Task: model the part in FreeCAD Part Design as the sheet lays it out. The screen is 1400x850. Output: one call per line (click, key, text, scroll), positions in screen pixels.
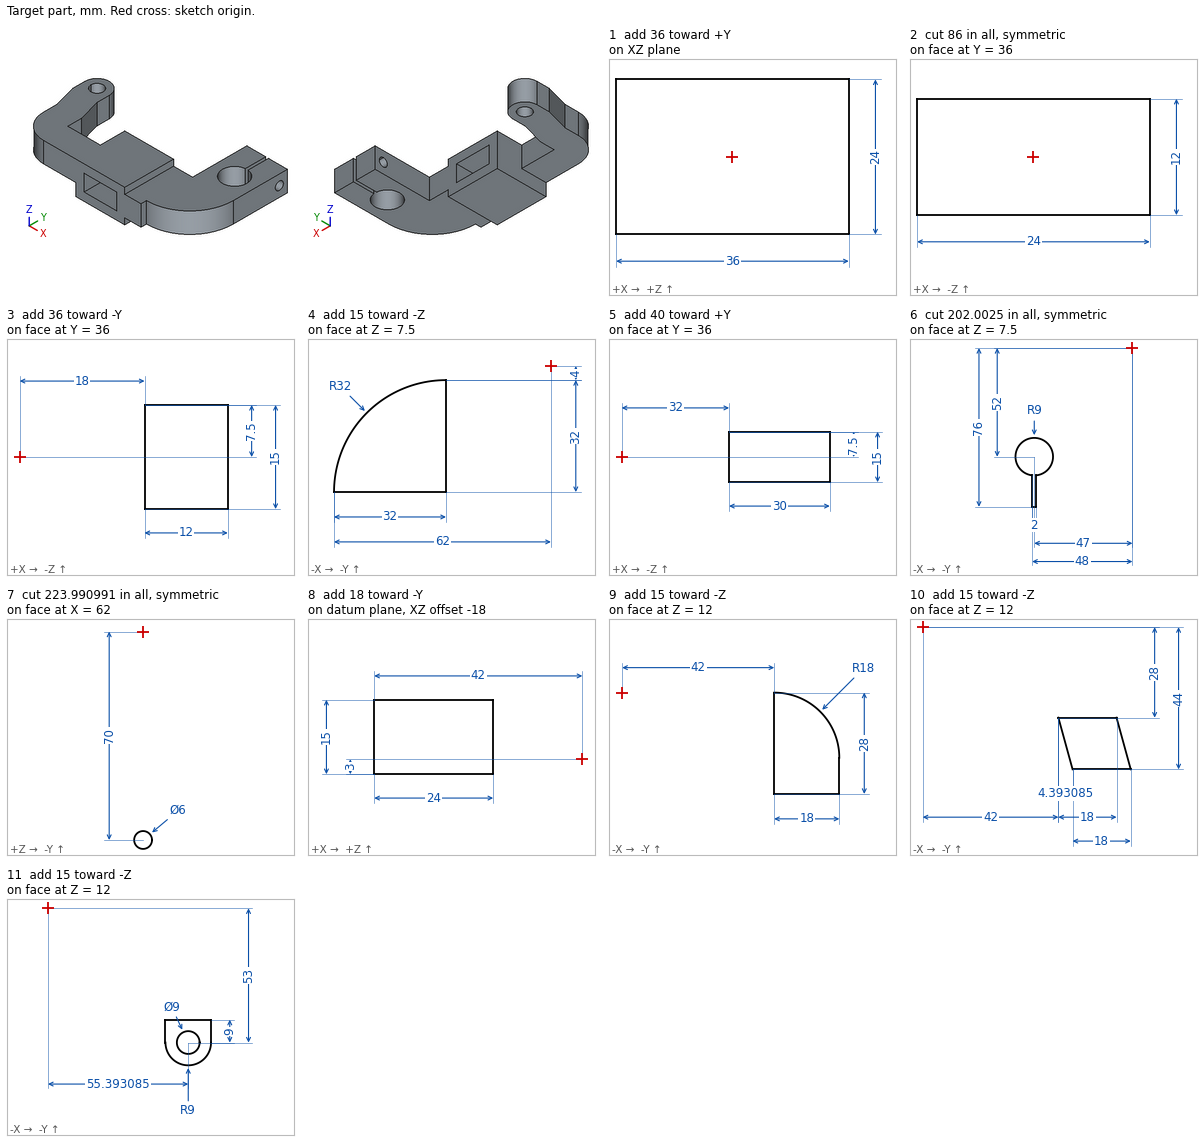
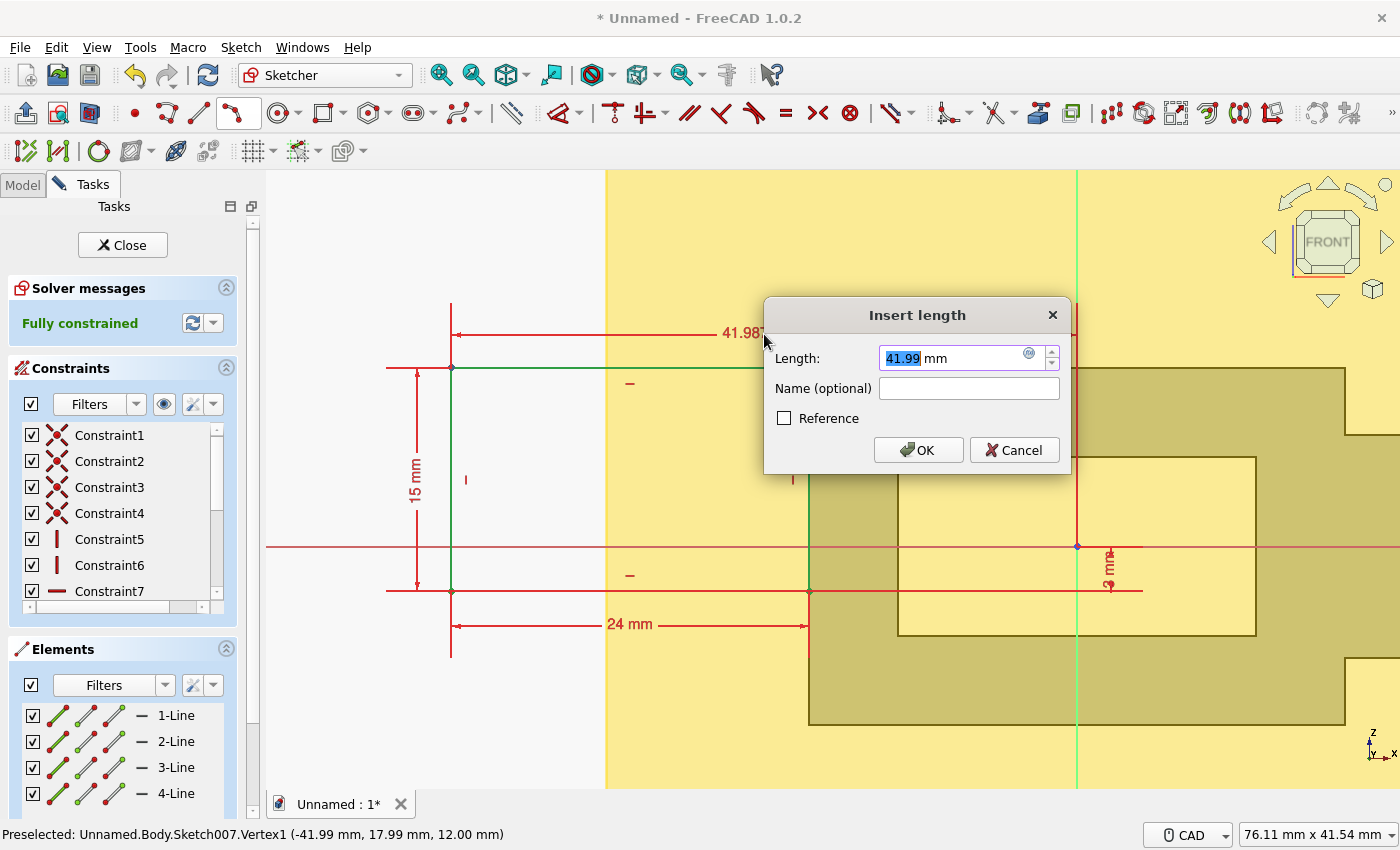
text(42)
key(Return)
key(Escape)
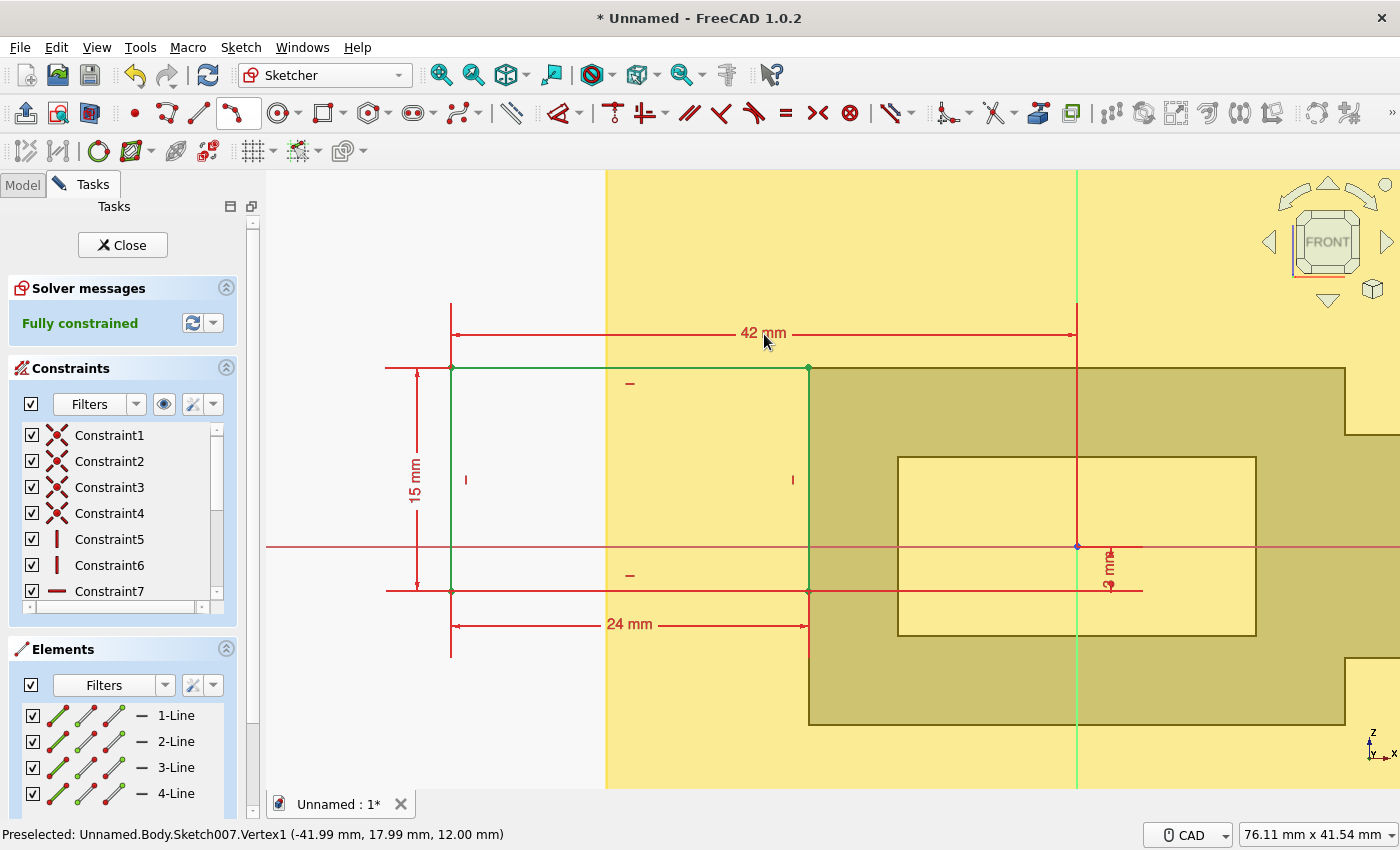
click(123, 245)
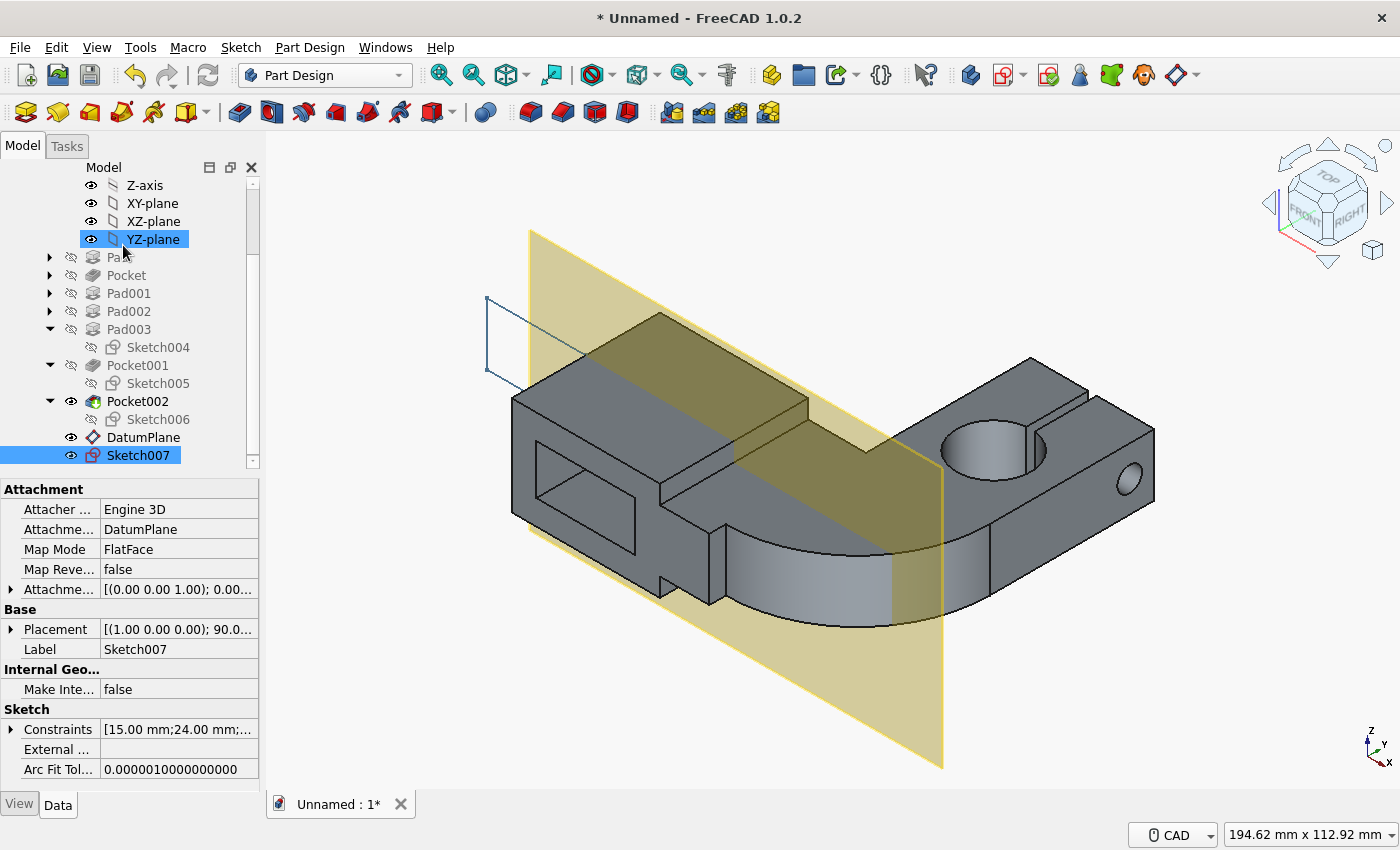
click(26, 112)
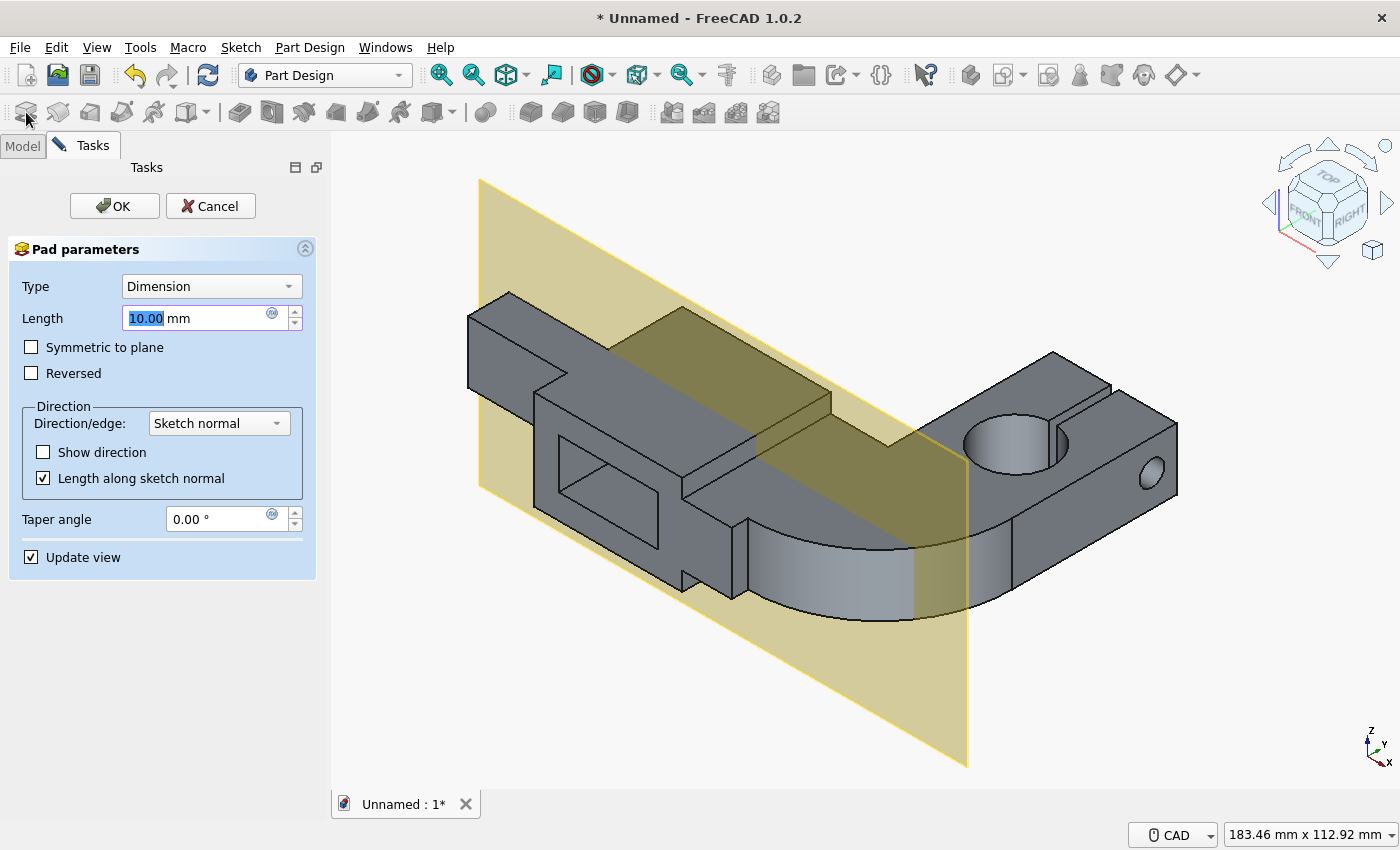
text(18)
key(Tab)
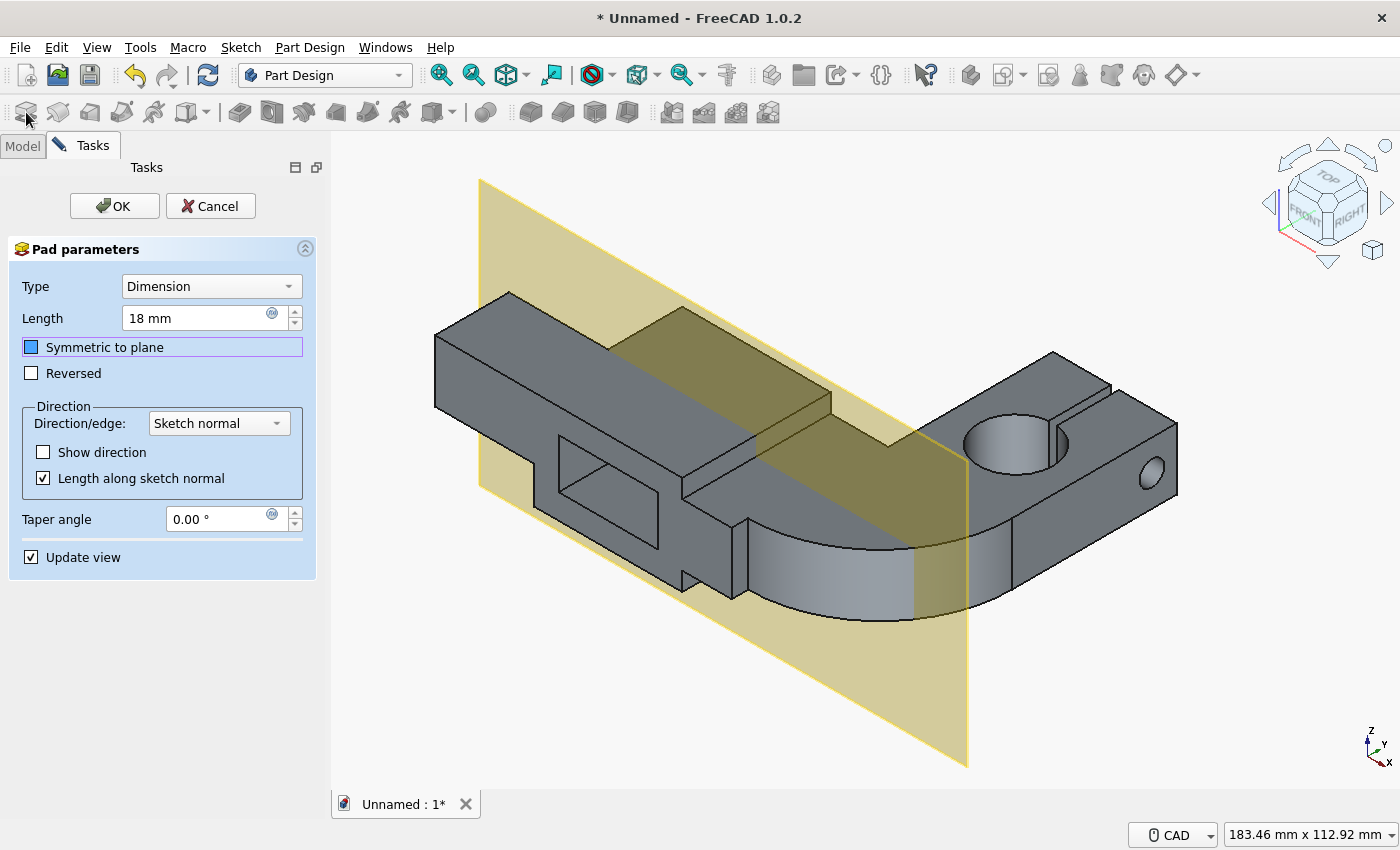
click(115, 206)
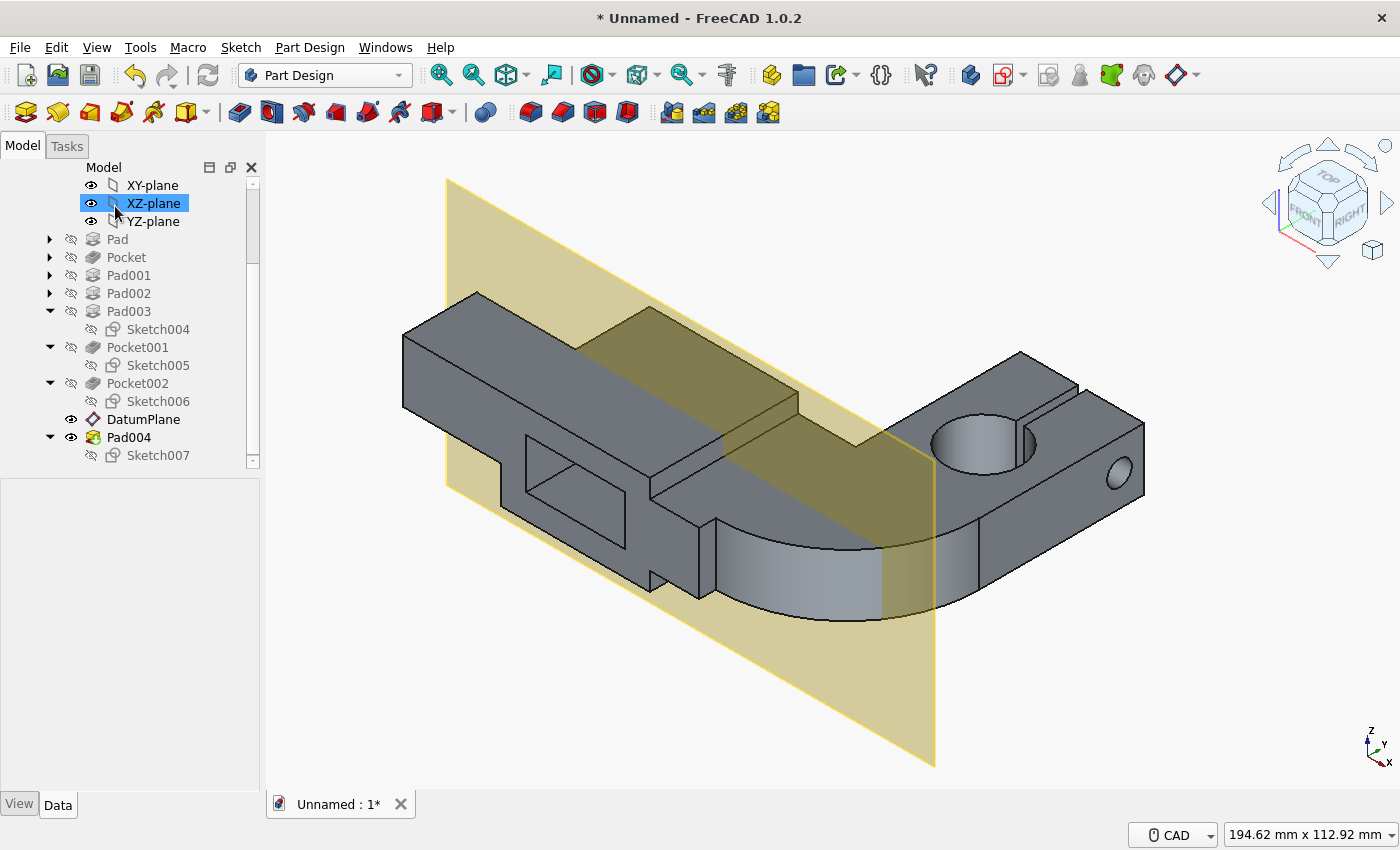
click(116, 419)
key(space)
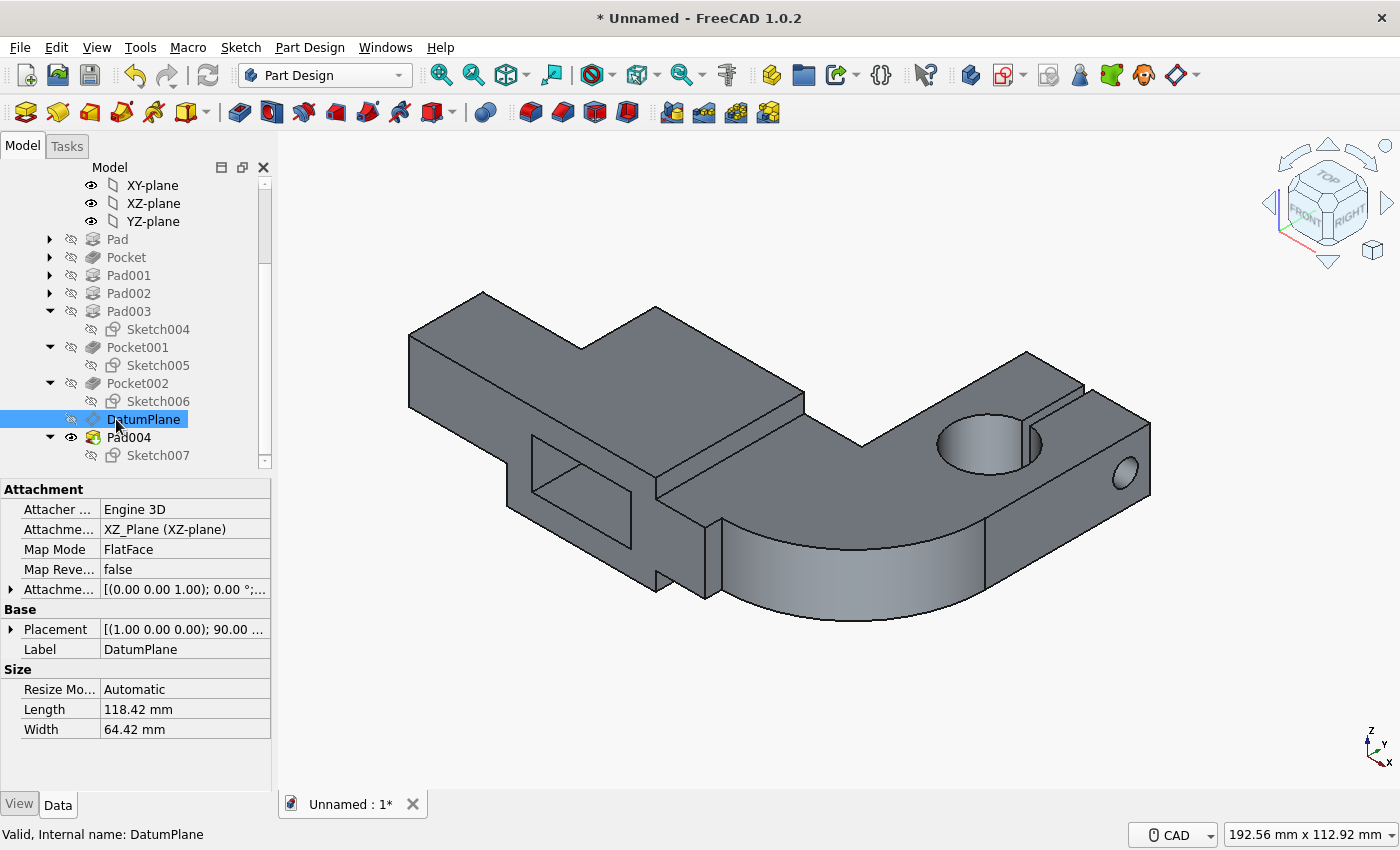
click(642, 383)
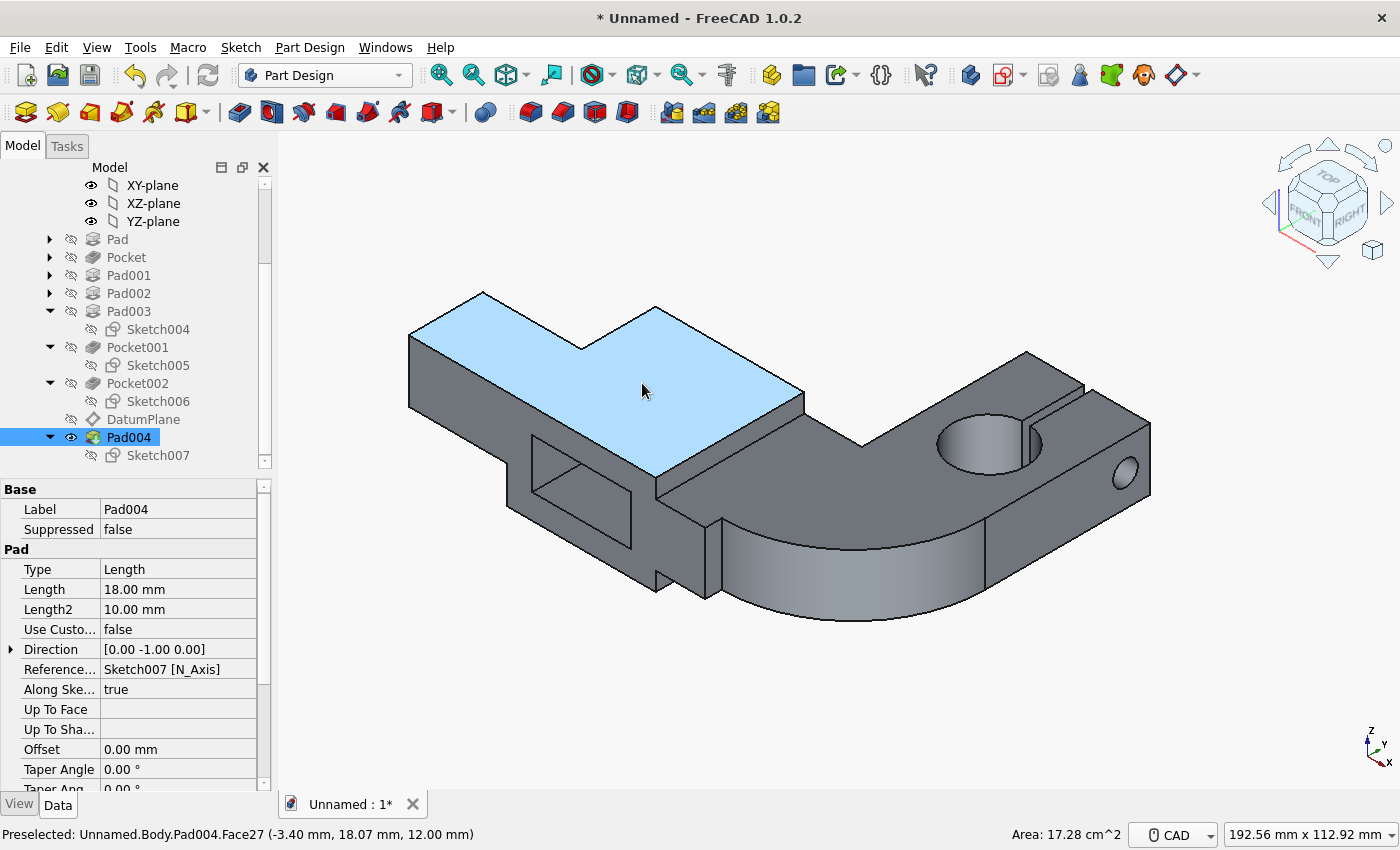
click(1004, 76)